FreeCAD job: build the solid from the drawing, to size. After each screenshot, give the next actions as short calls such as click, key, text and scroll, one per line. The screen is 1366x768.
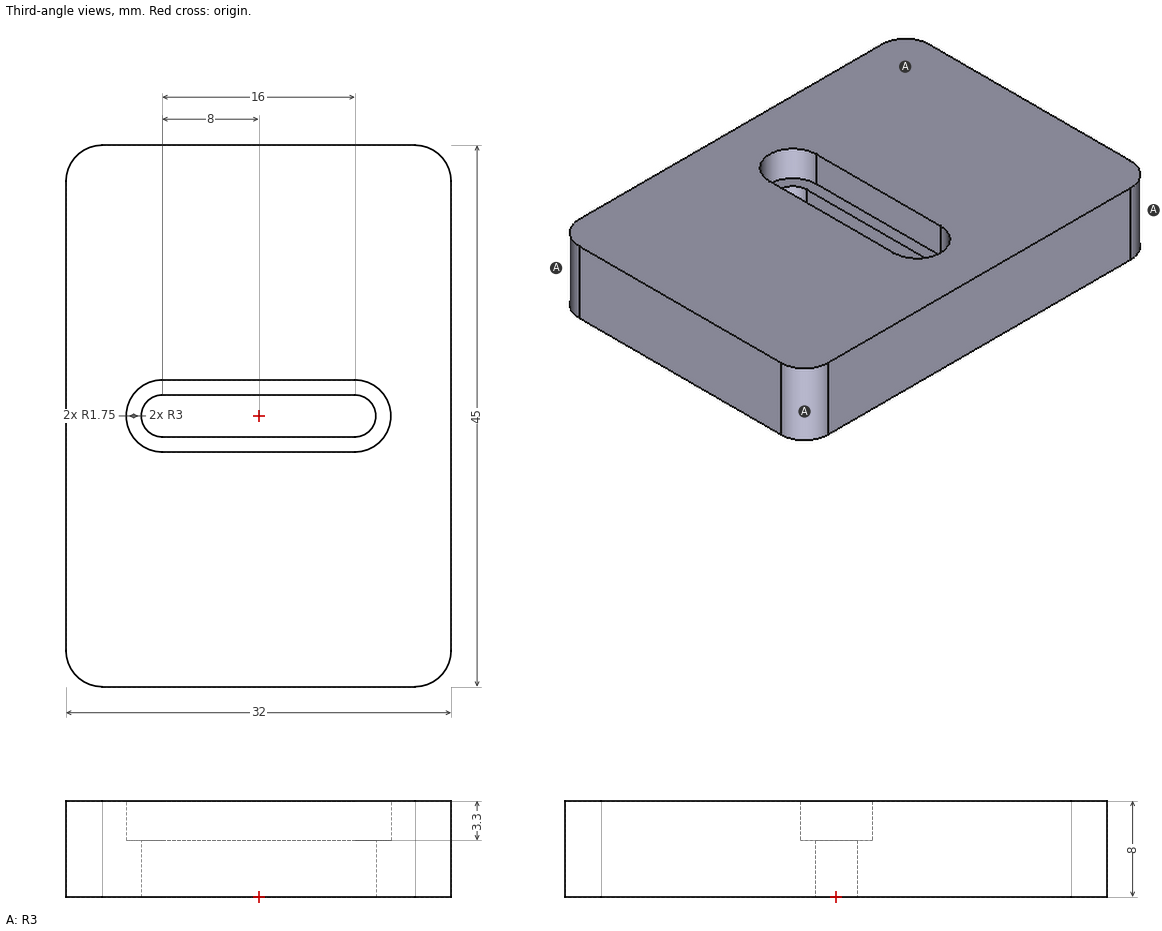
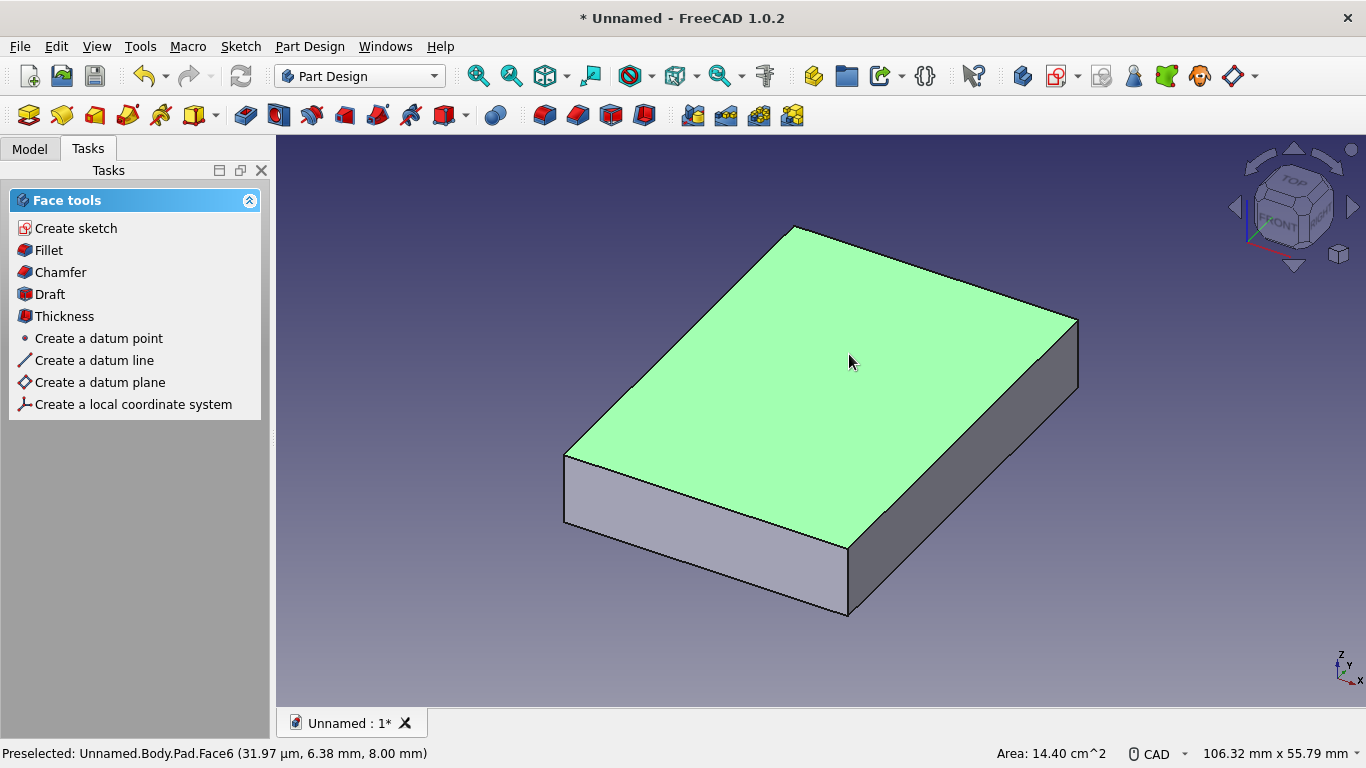
click(1056, 76)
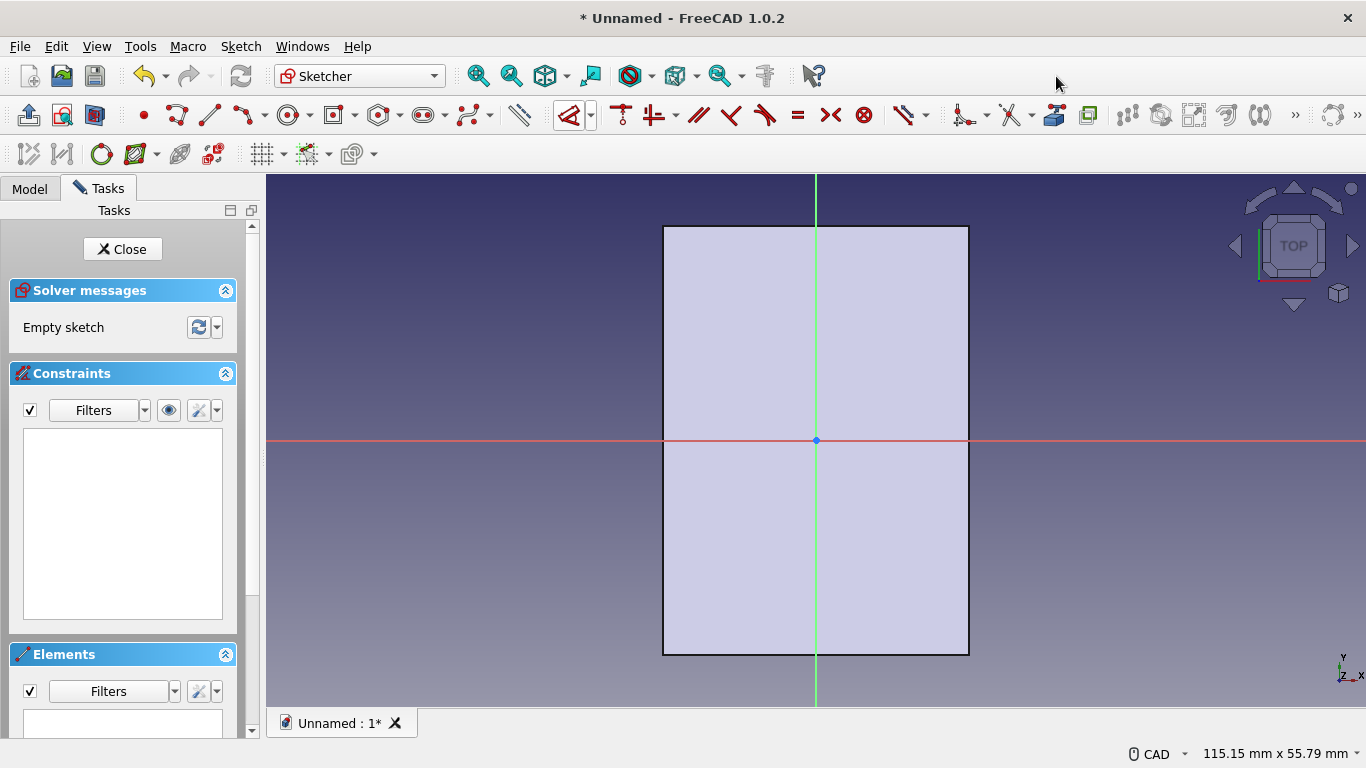
scroll(846, 440, up, 6)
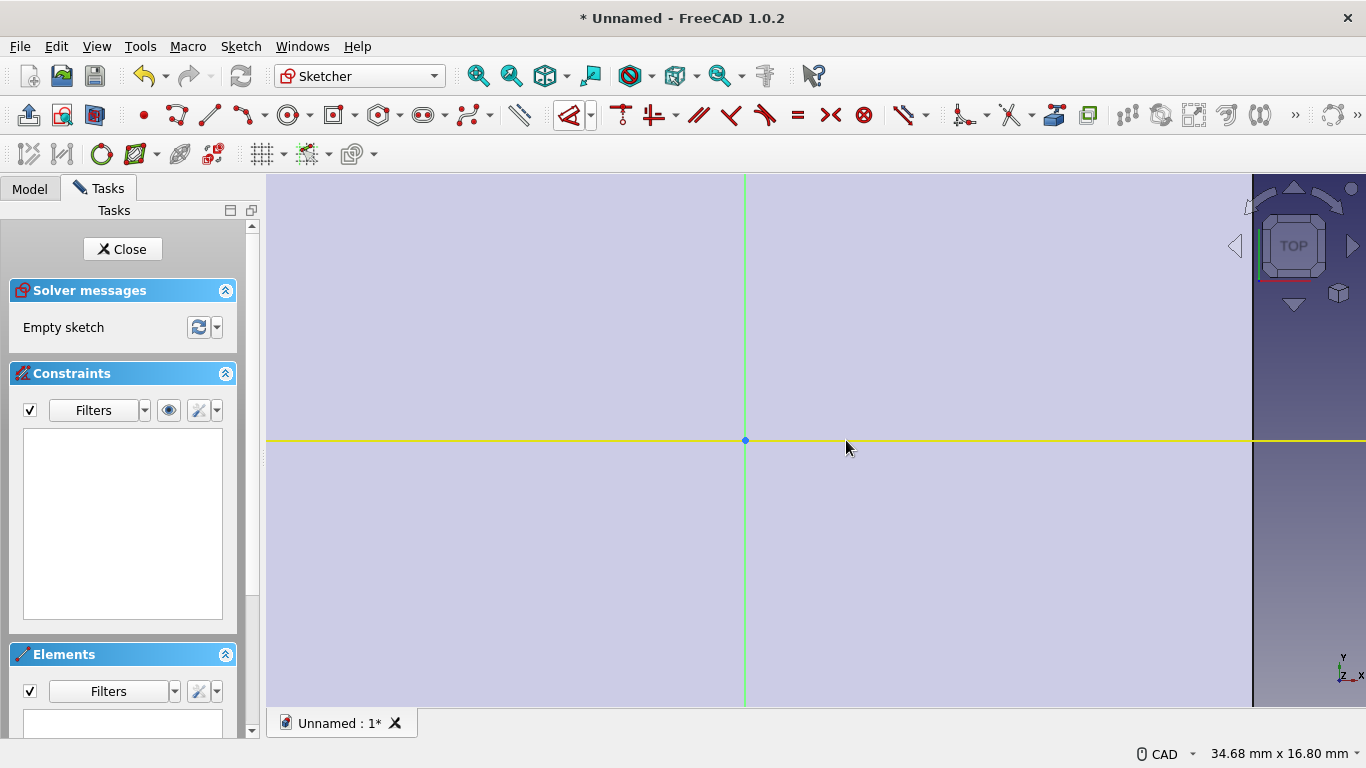
click(422, 116)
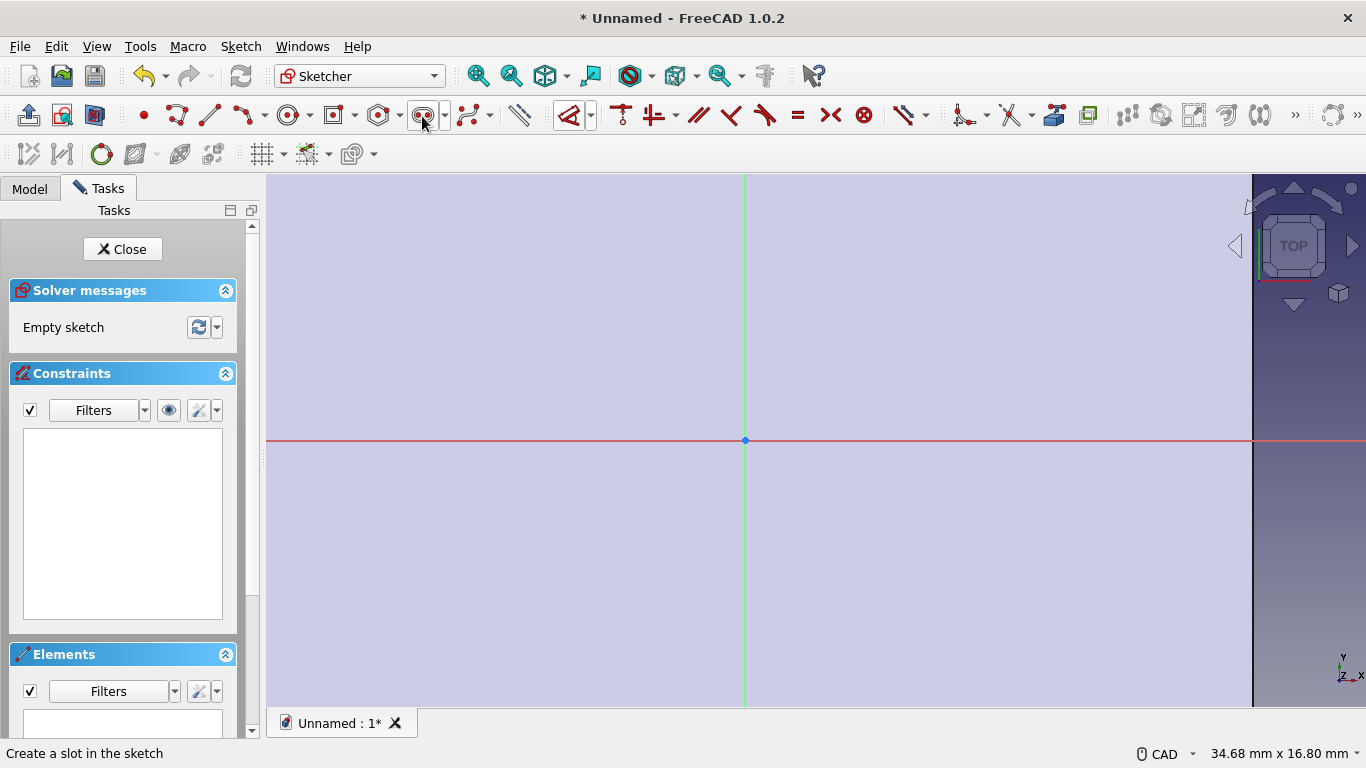
click(491, 440)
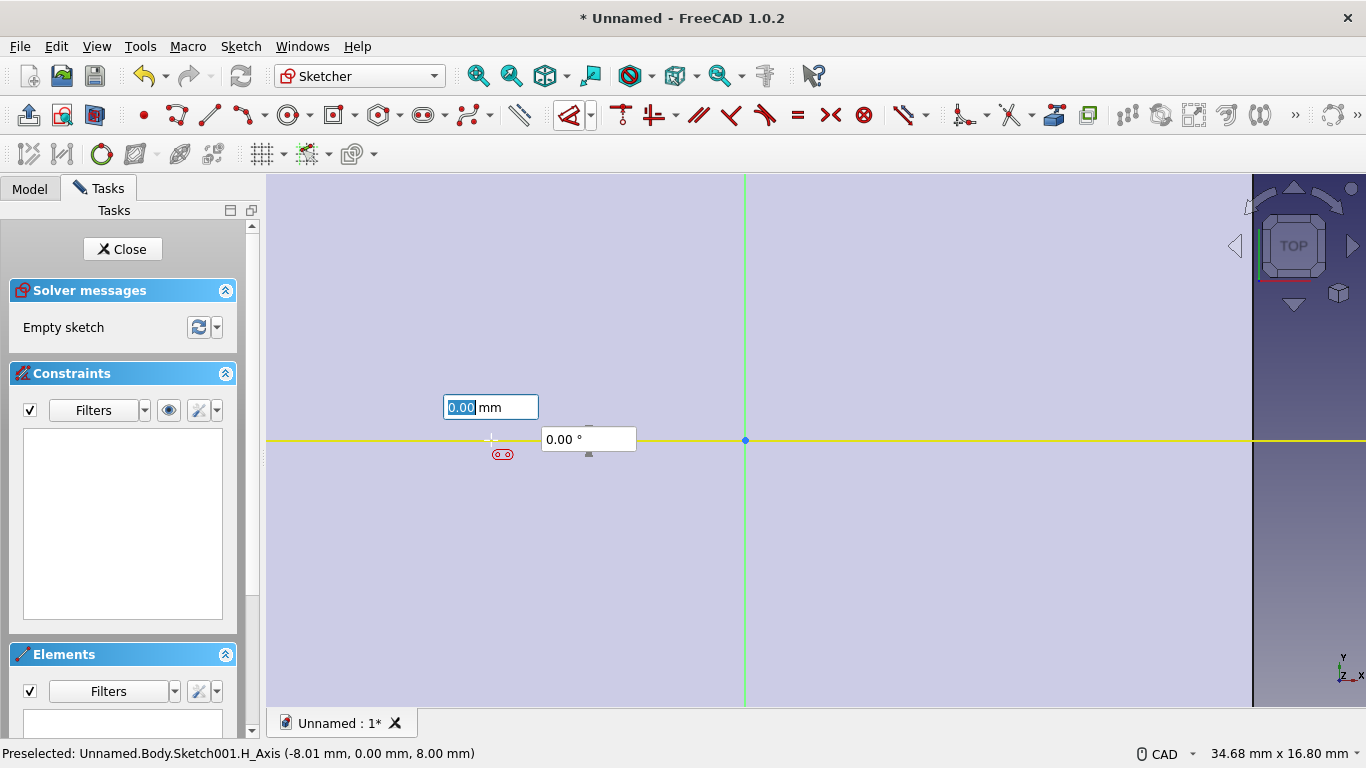
click(999, 432)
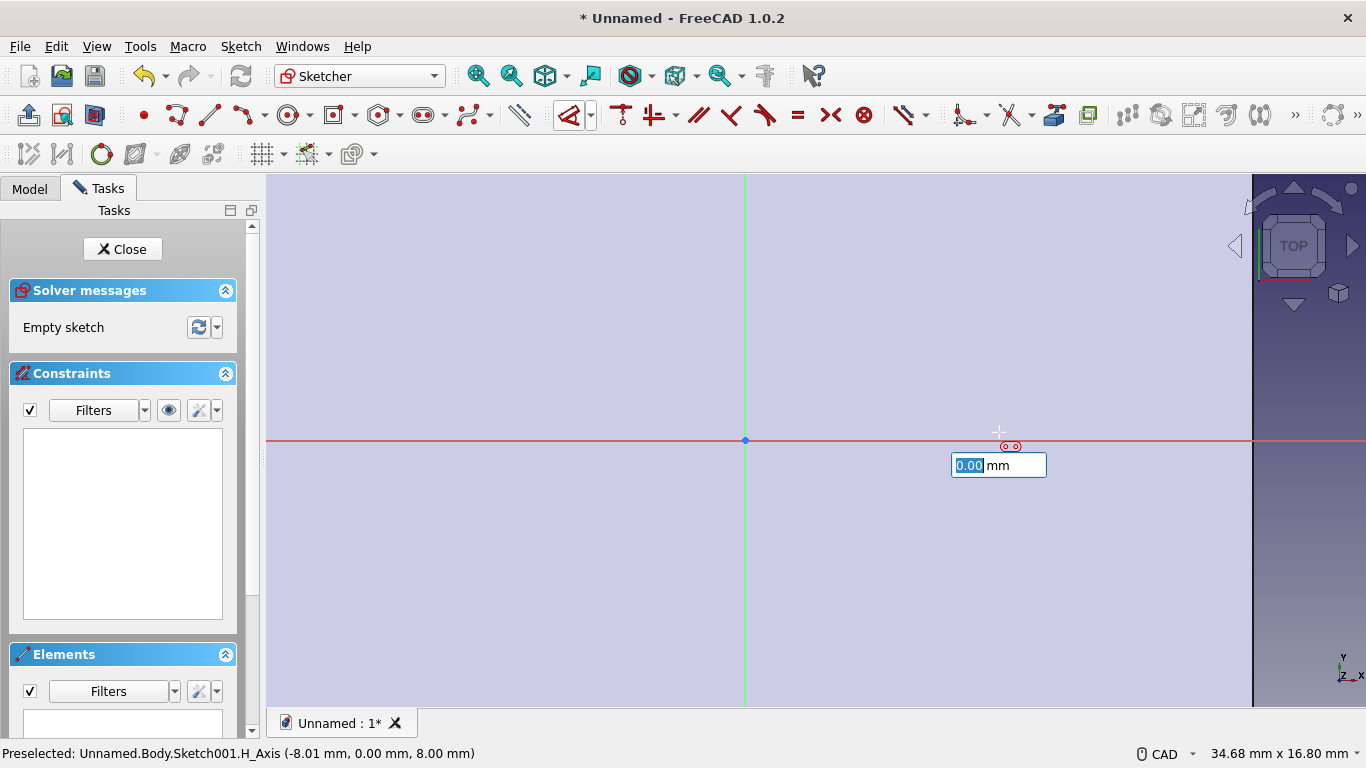
click(821, 385)
key(Escape)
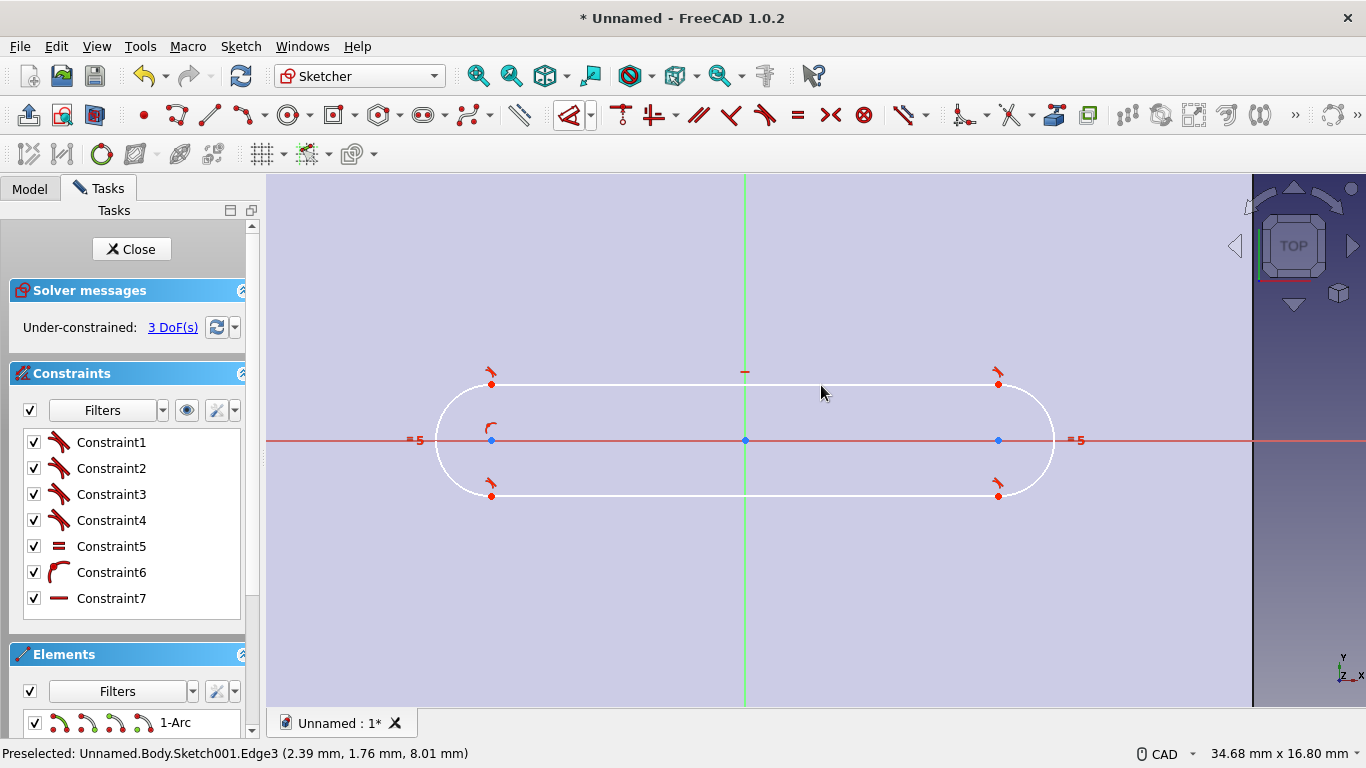
click(568, 116)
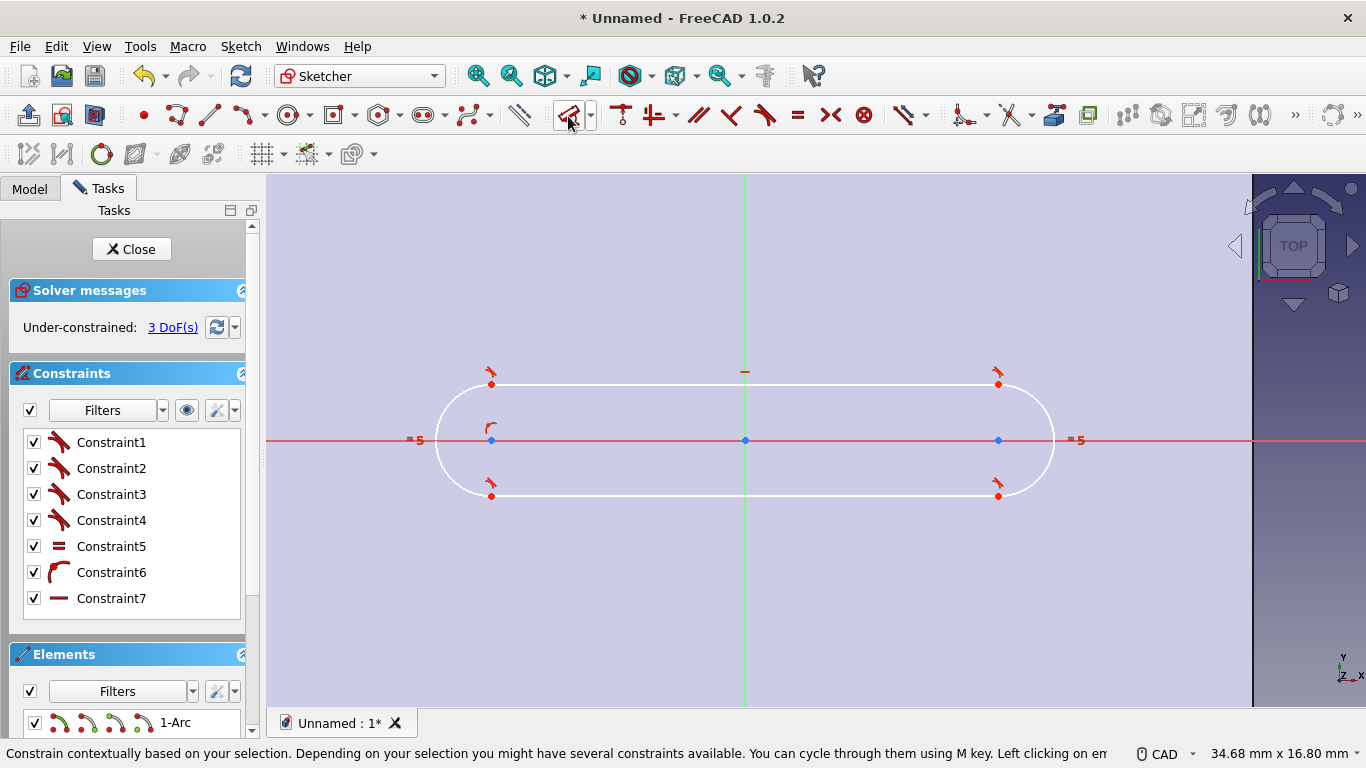
click(447, 408)
click(421, 389)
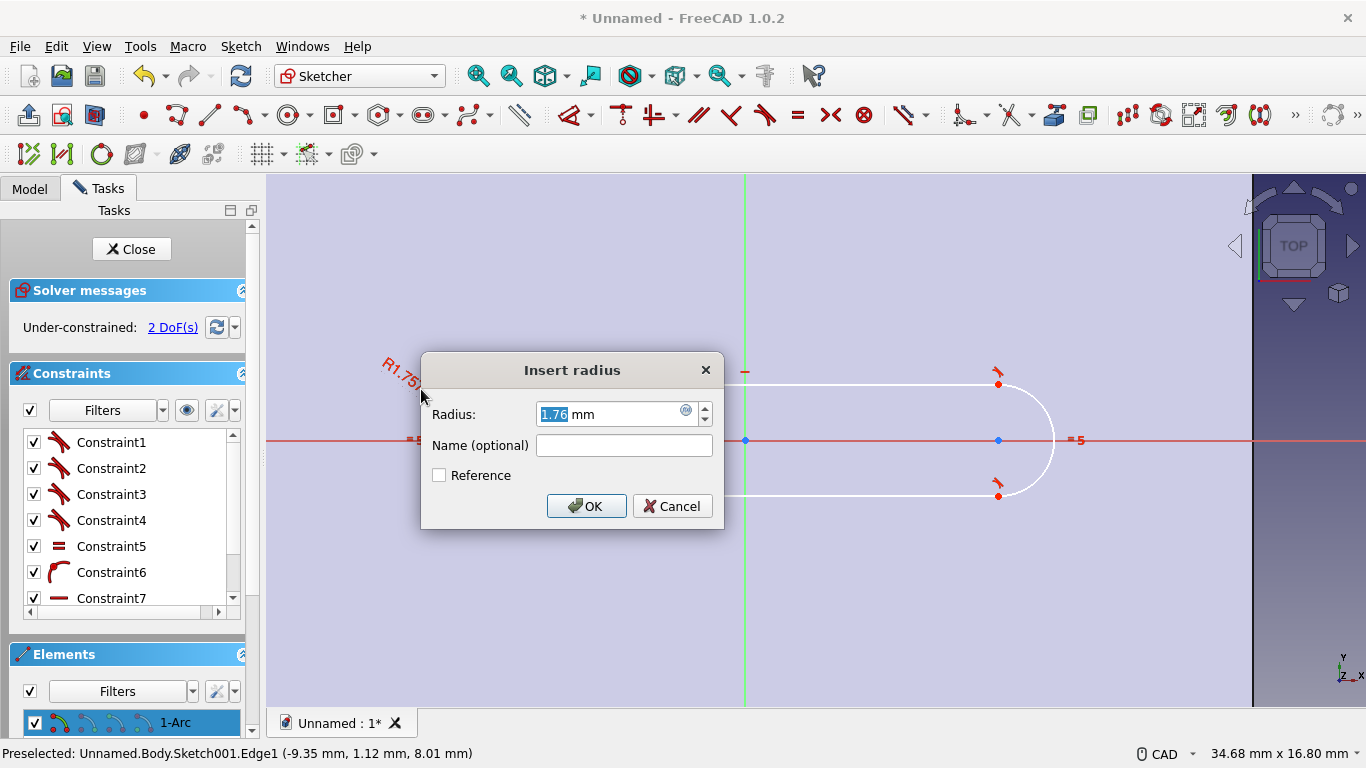
text(1.75)
key(Return)